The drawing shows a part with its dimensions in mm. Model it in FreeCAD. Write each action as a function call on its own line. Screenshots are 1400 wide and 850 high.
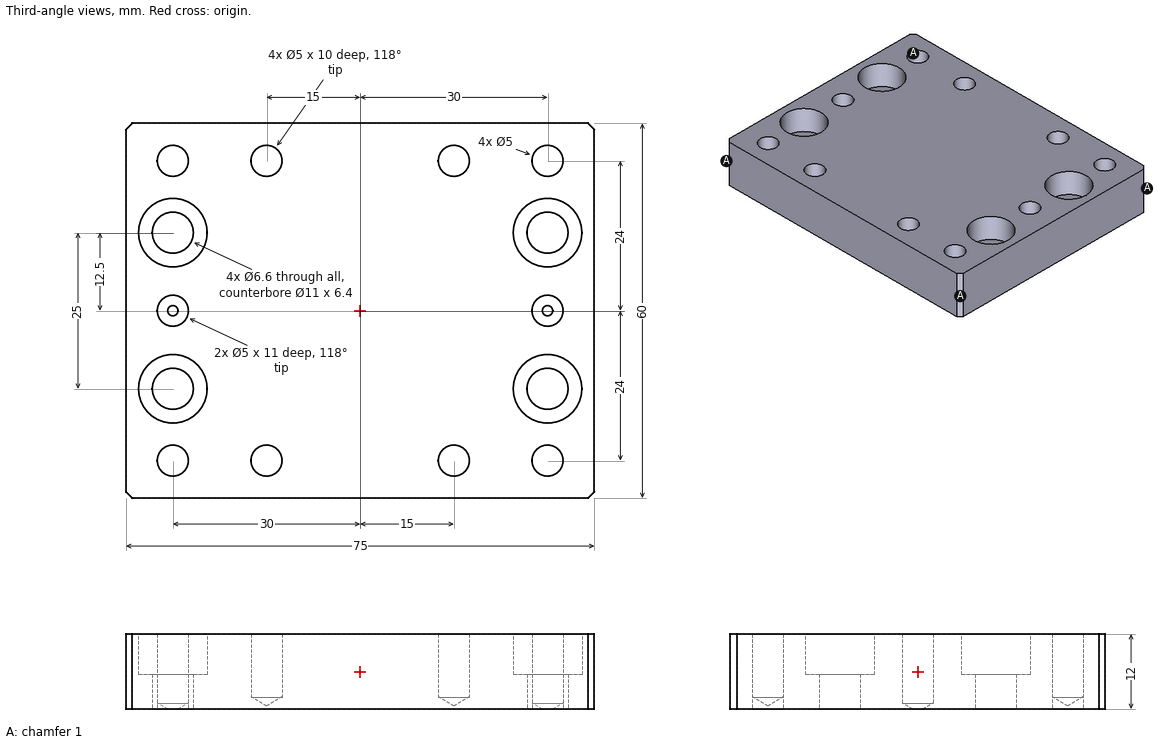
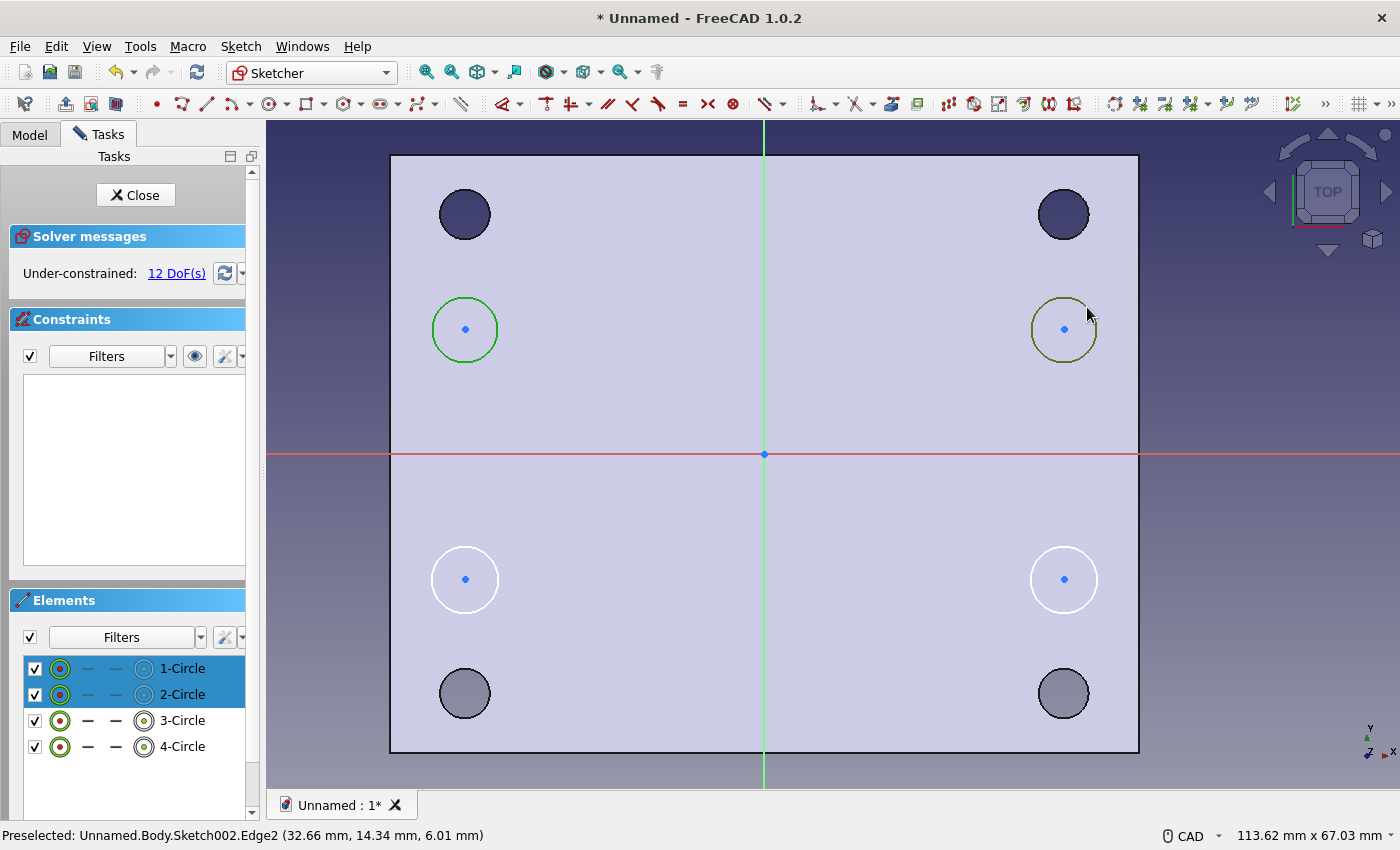
click(488, 556)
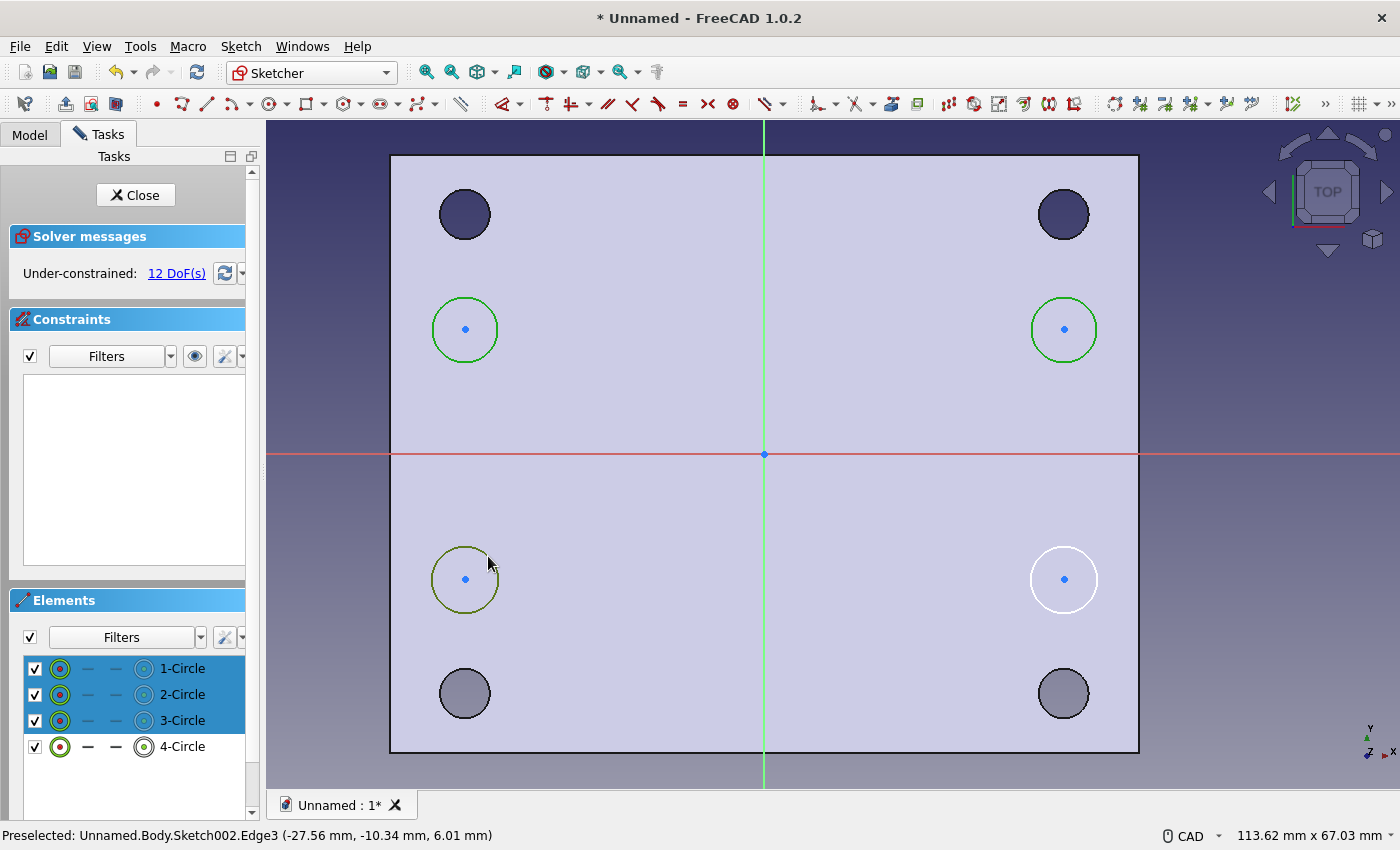
click(1087, 556)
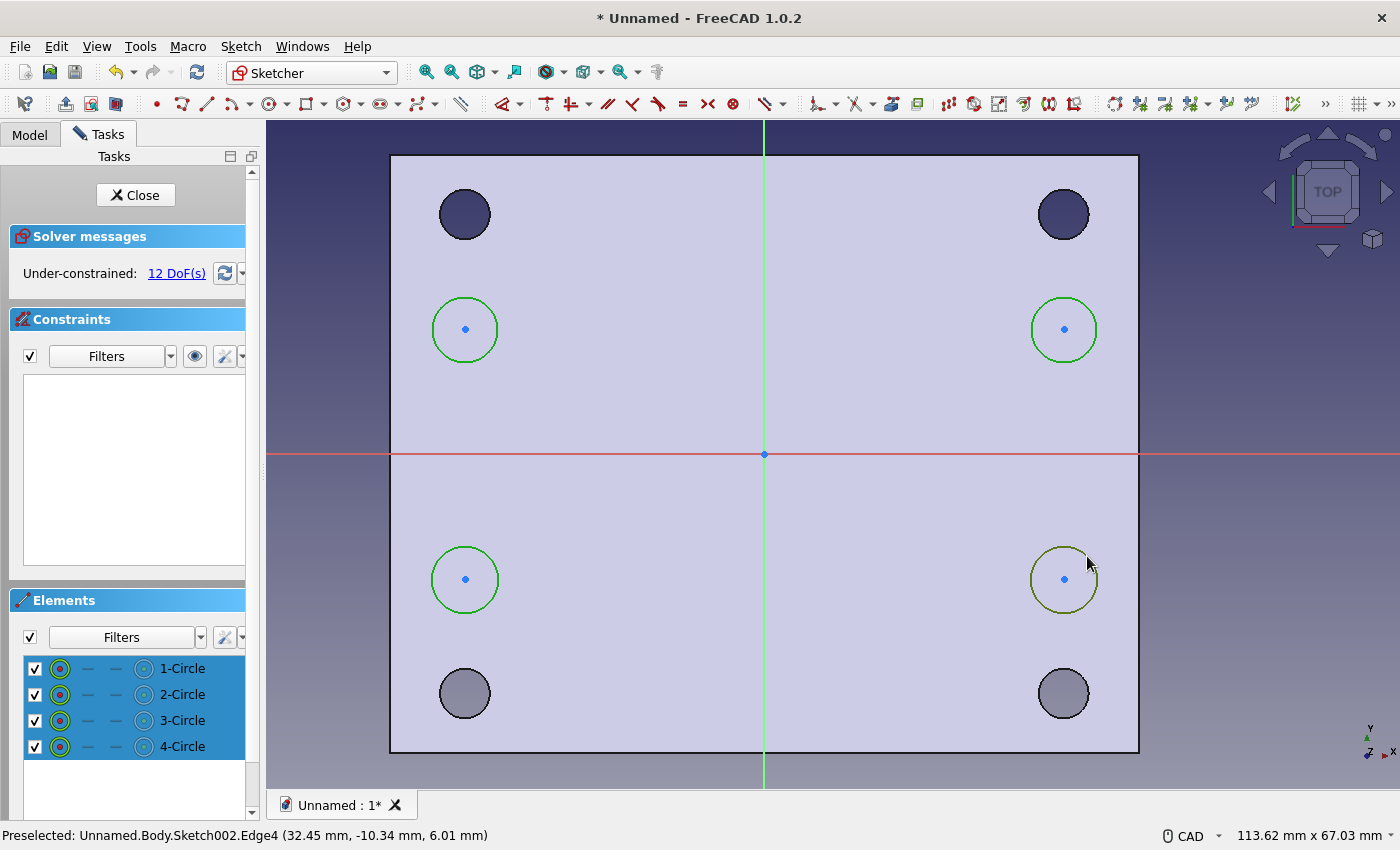
click(683, 104)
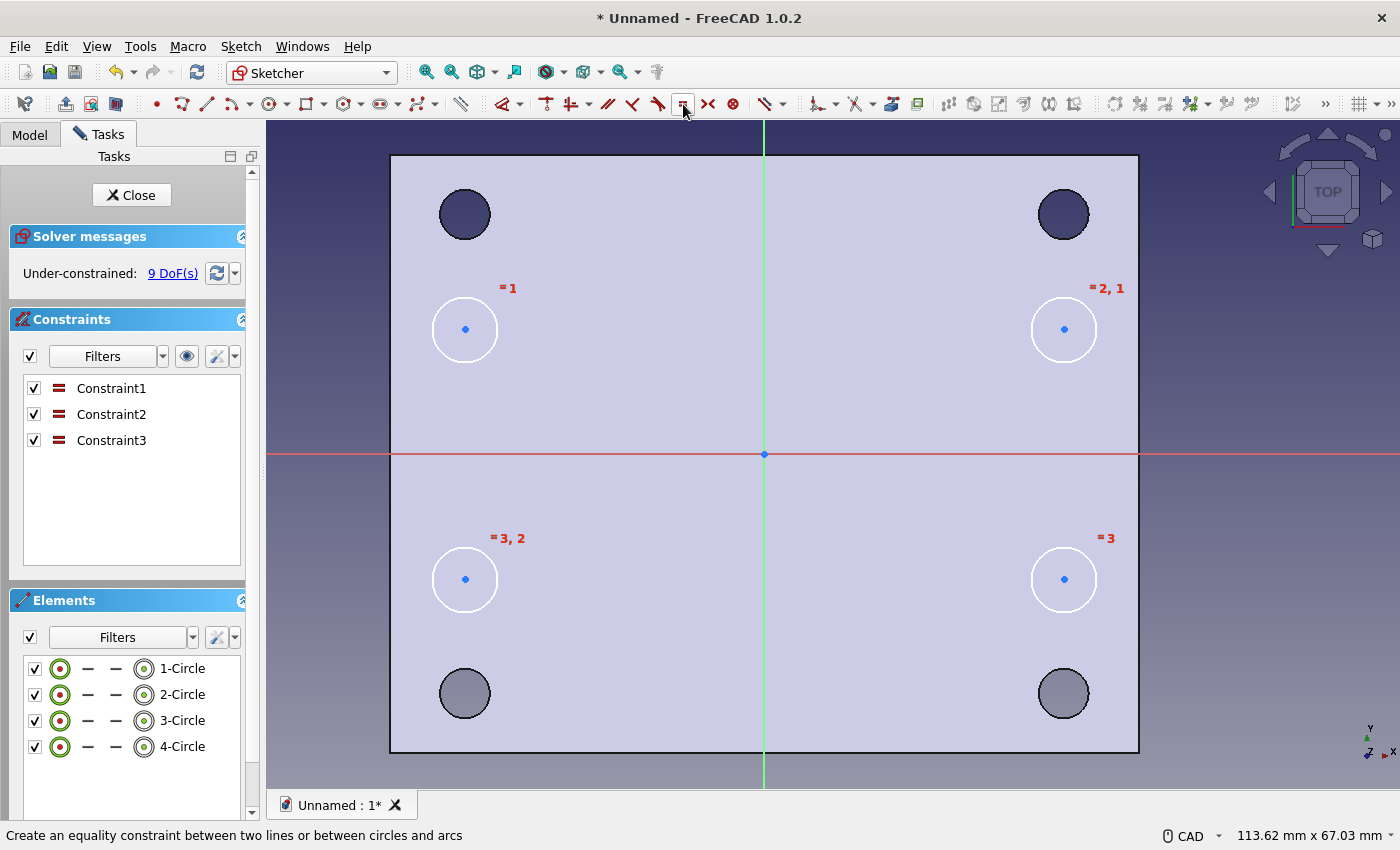
key(d)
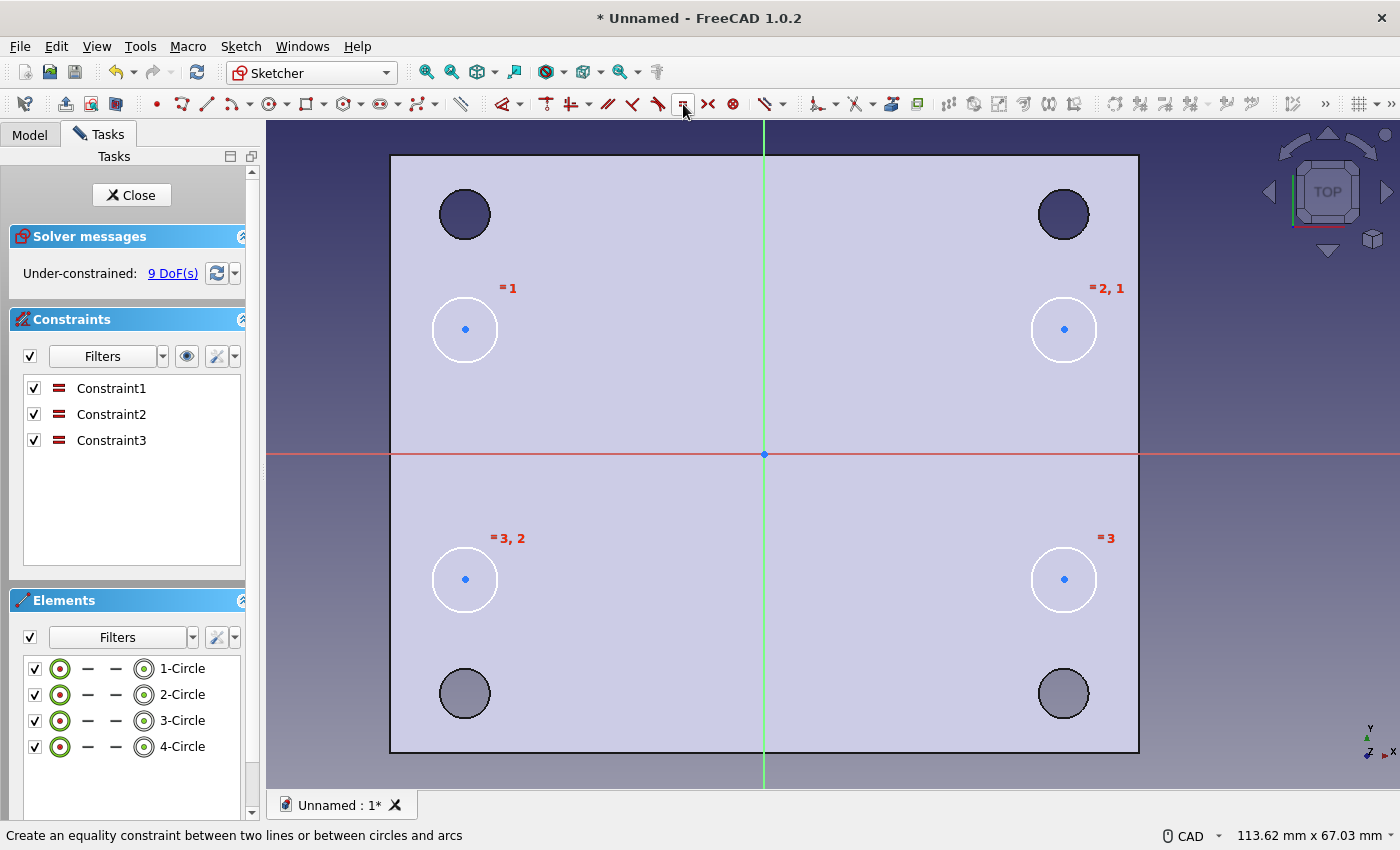
click(488, 307)
click(511, 284)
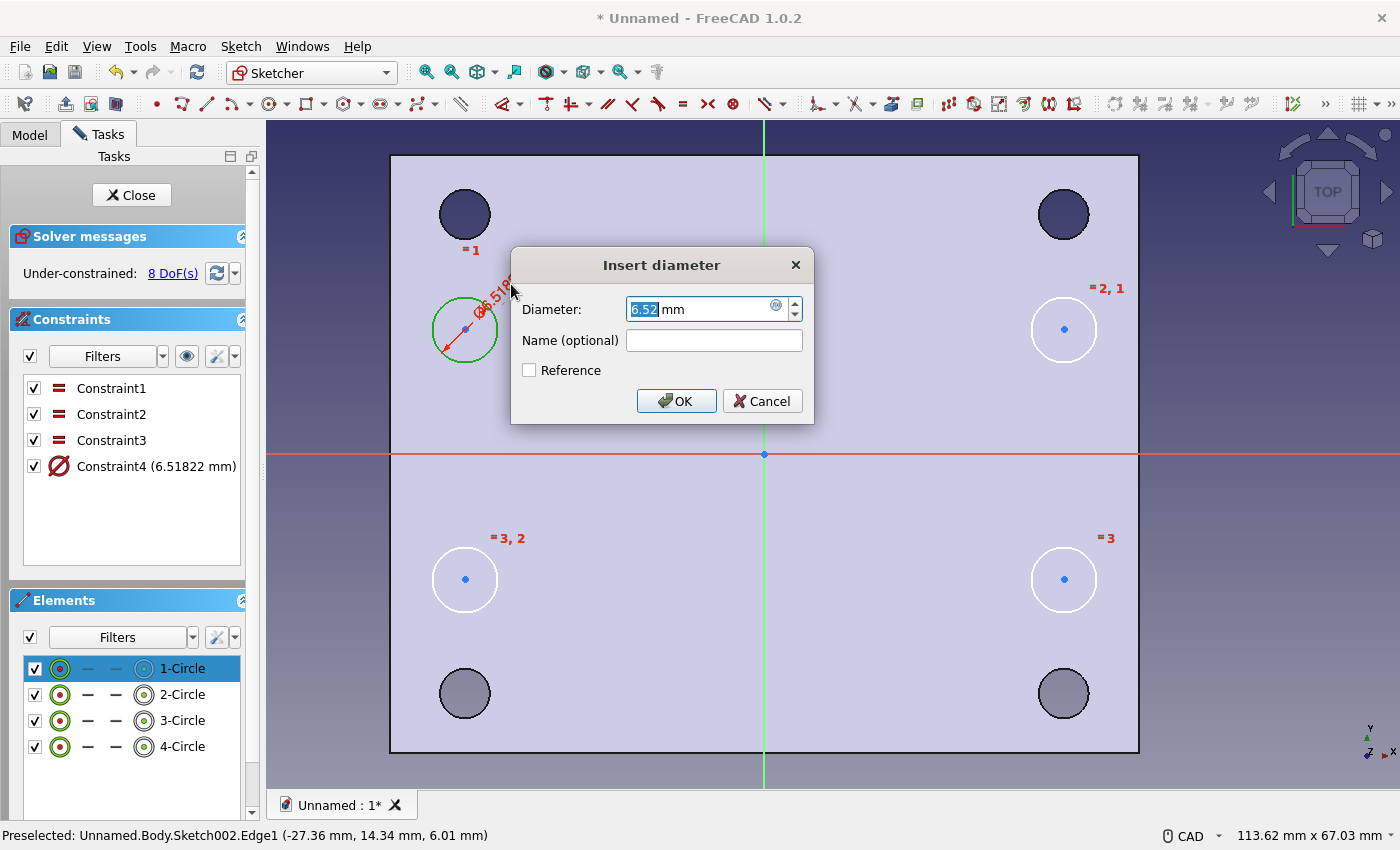
text(6.6)
key(Return)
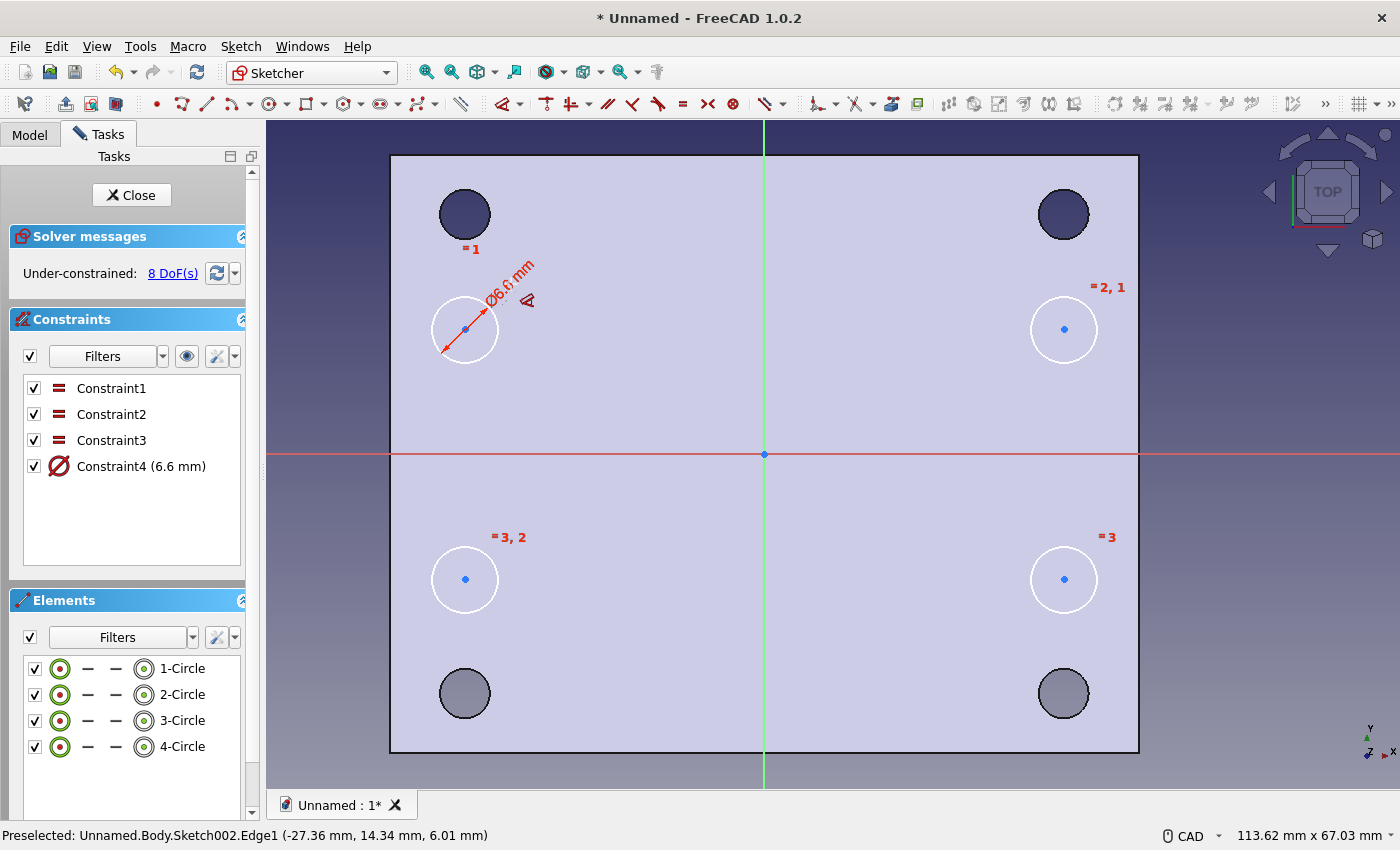
click(465, 330)
click(615, 296)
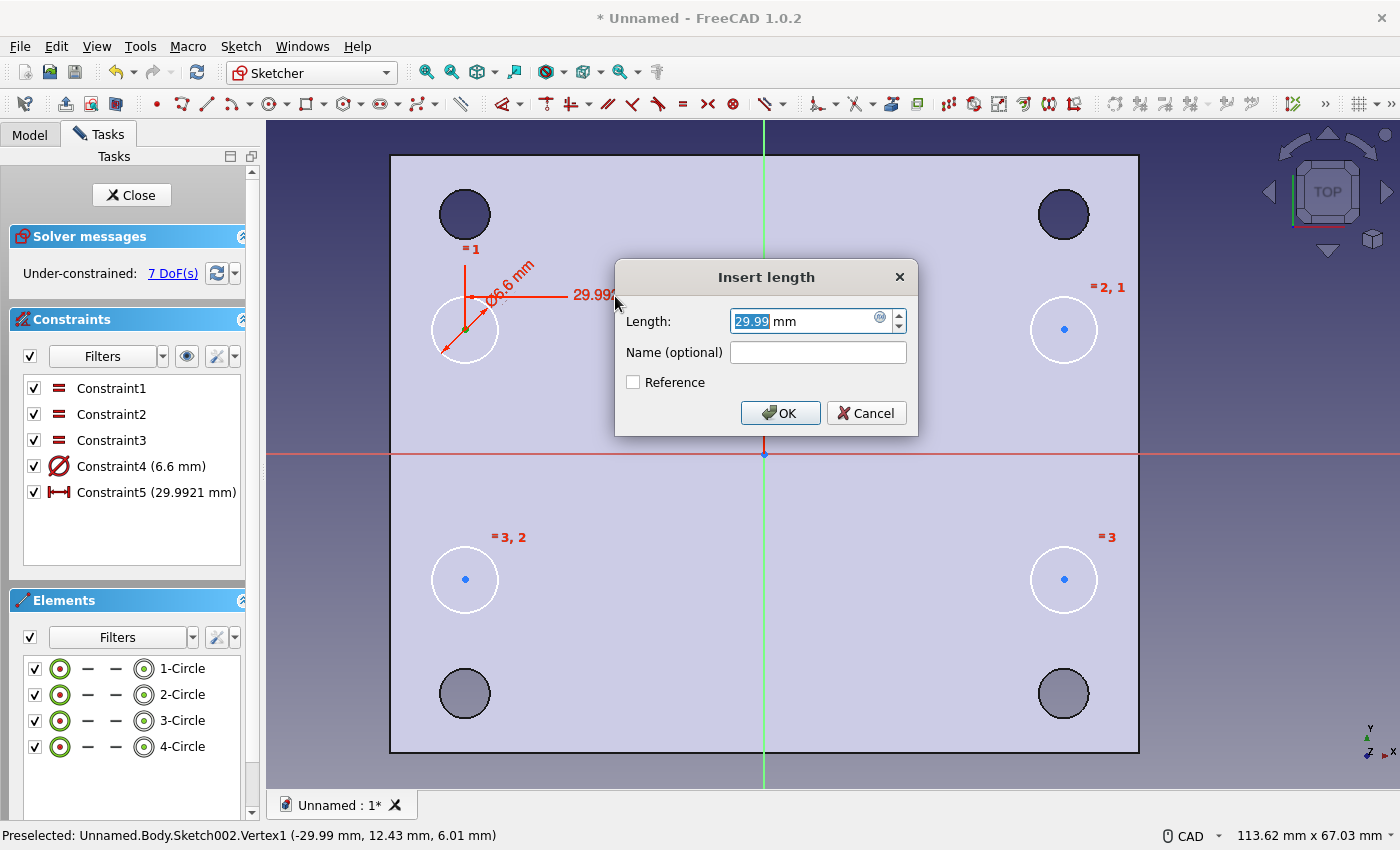
text(30)
key(Return)